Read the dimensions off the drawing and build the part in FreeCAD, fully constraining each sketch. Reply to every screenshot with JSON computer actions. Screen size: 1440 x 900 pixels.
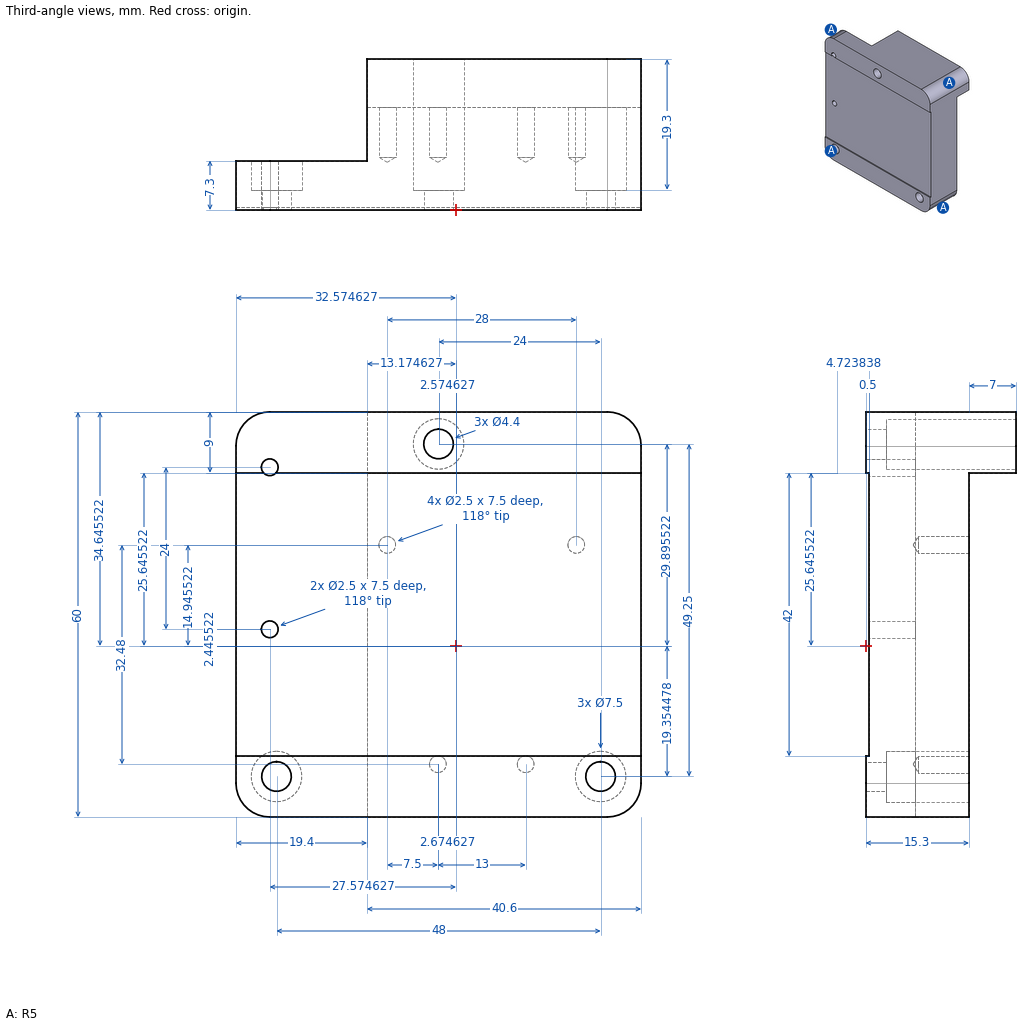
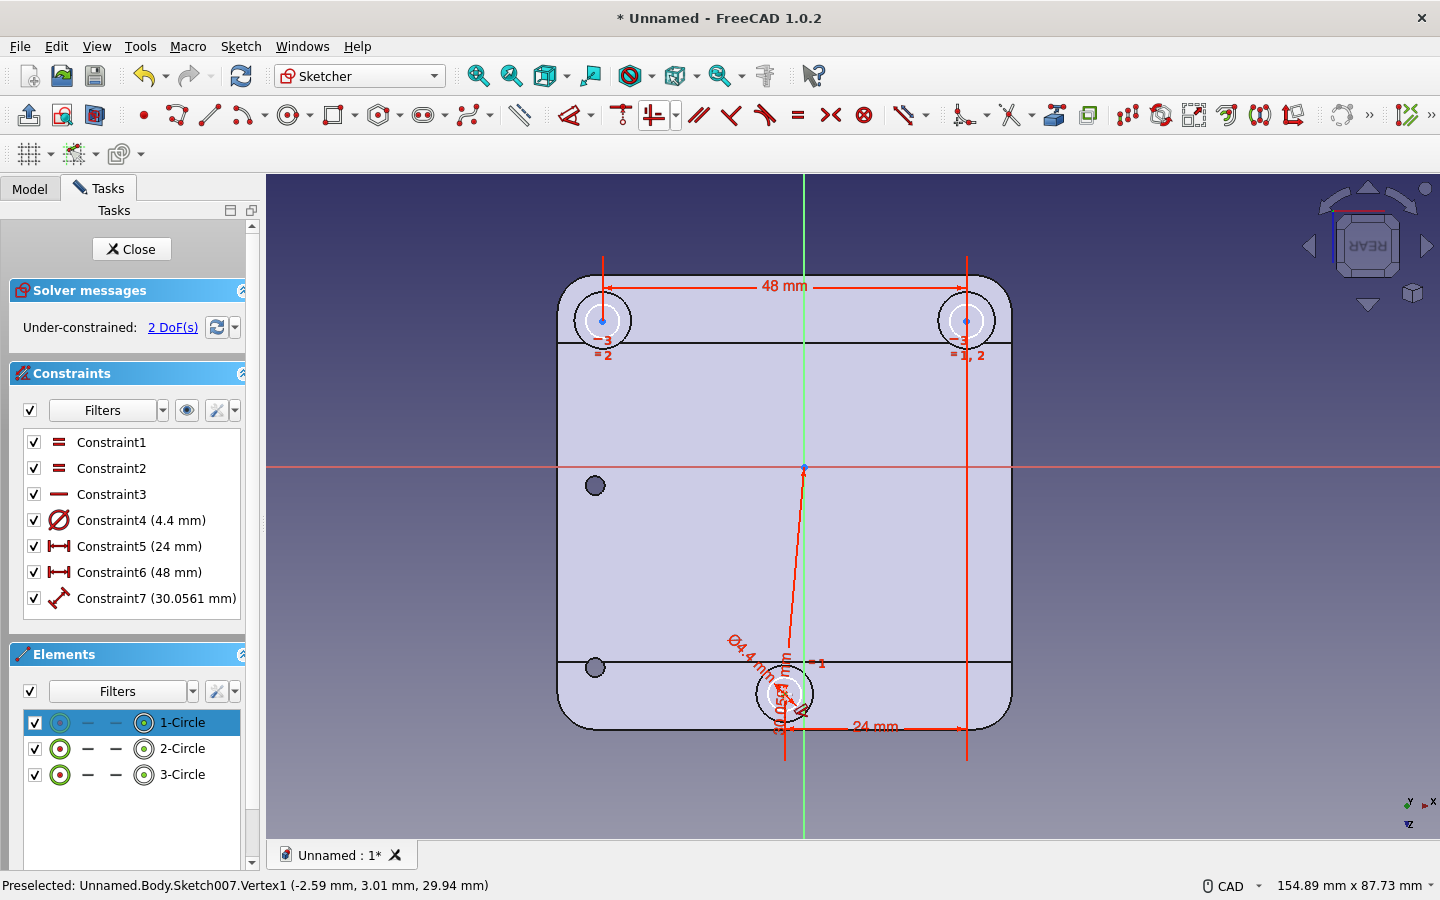
{"action": "left_click", "coordinate": [967, 321]}
{"action": "left_click", "coordinate": [1001, 508]}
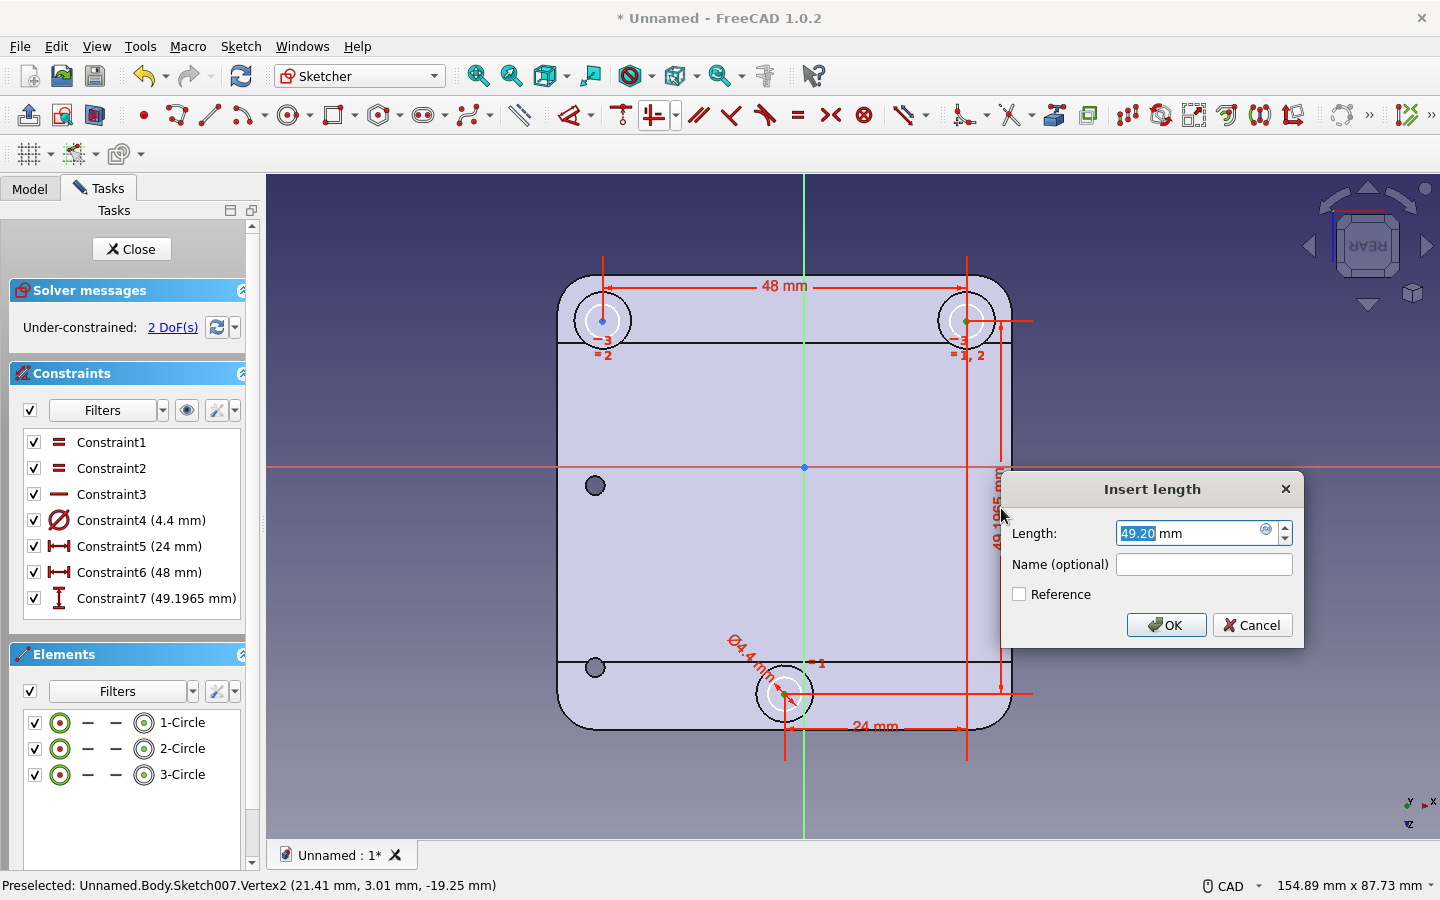
{"action": "type", "text": "49.25"}
{"action": "key", "text": "Return"}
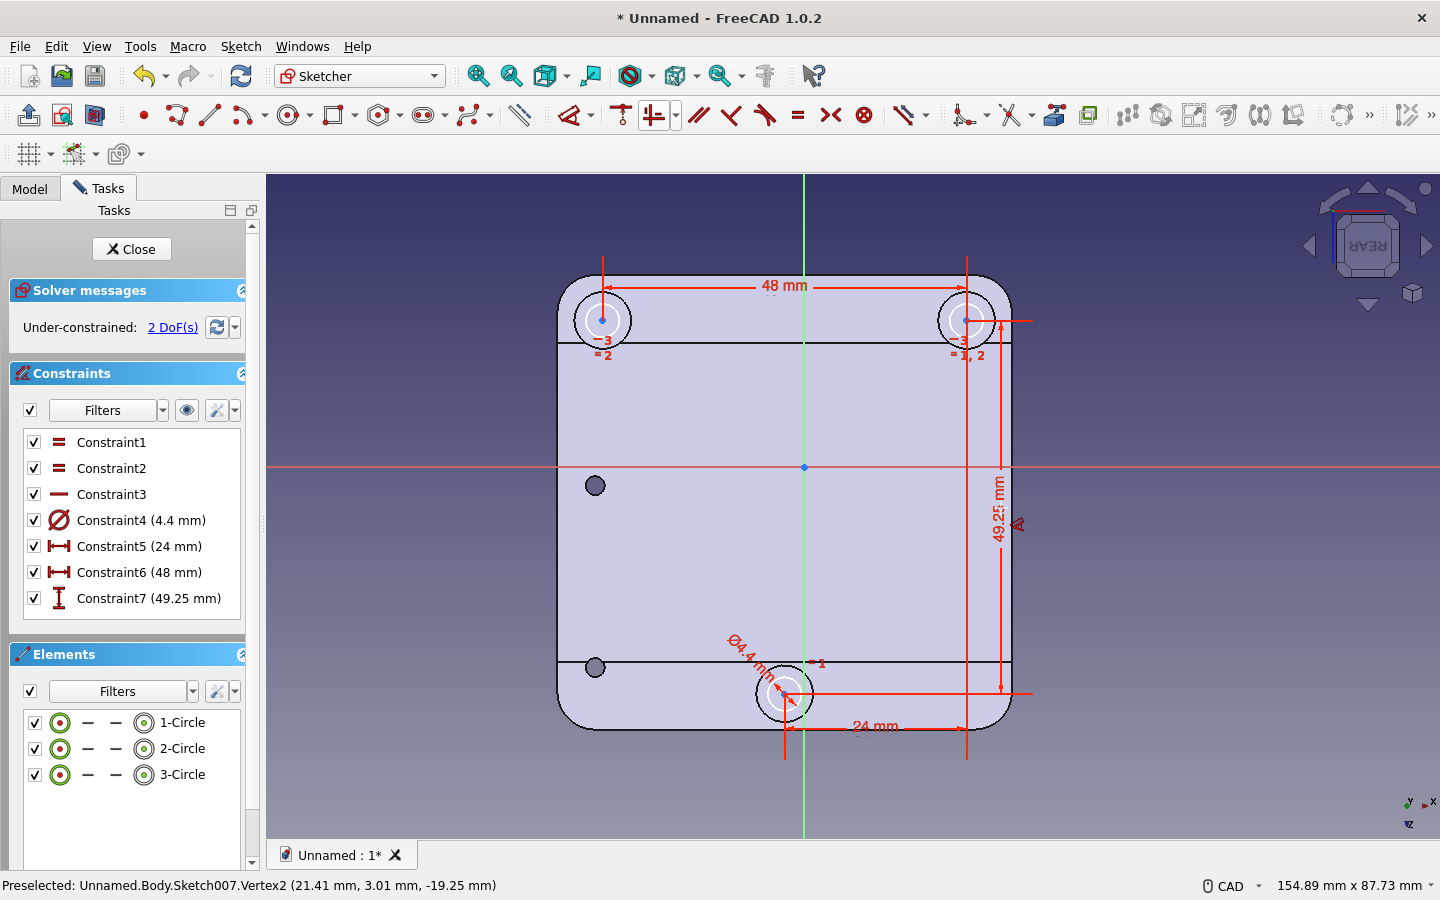
{"action": "scroll", "coordinate": [785, 694], "scroll_direction": "up", "scroll_amount": 4}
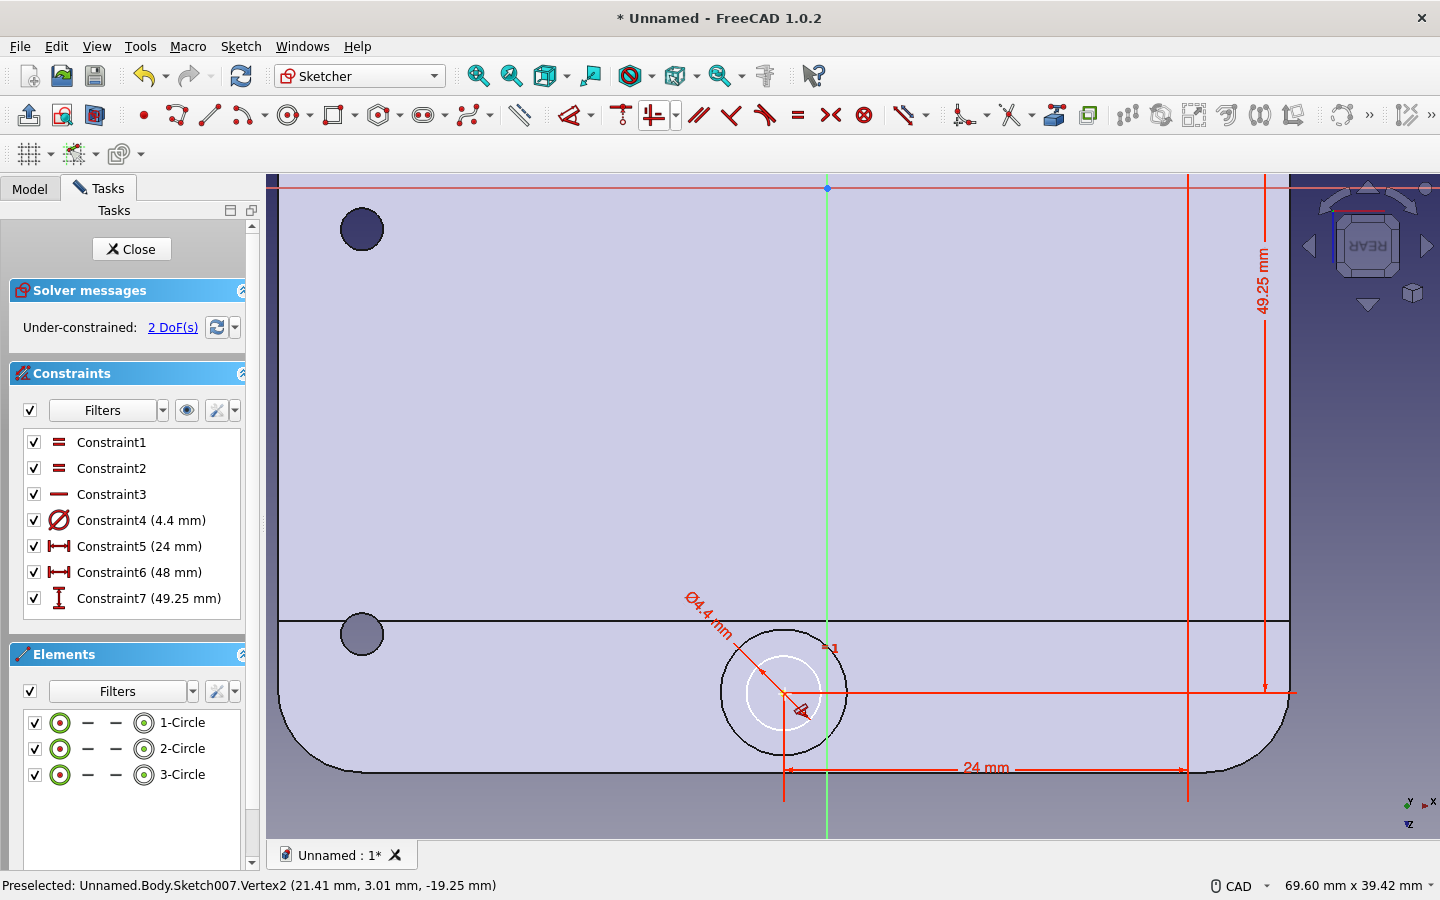
{"action": "left_click", "coordinate": [784, 693]}
{"action": "left_click", "coordinate": [805, 751]}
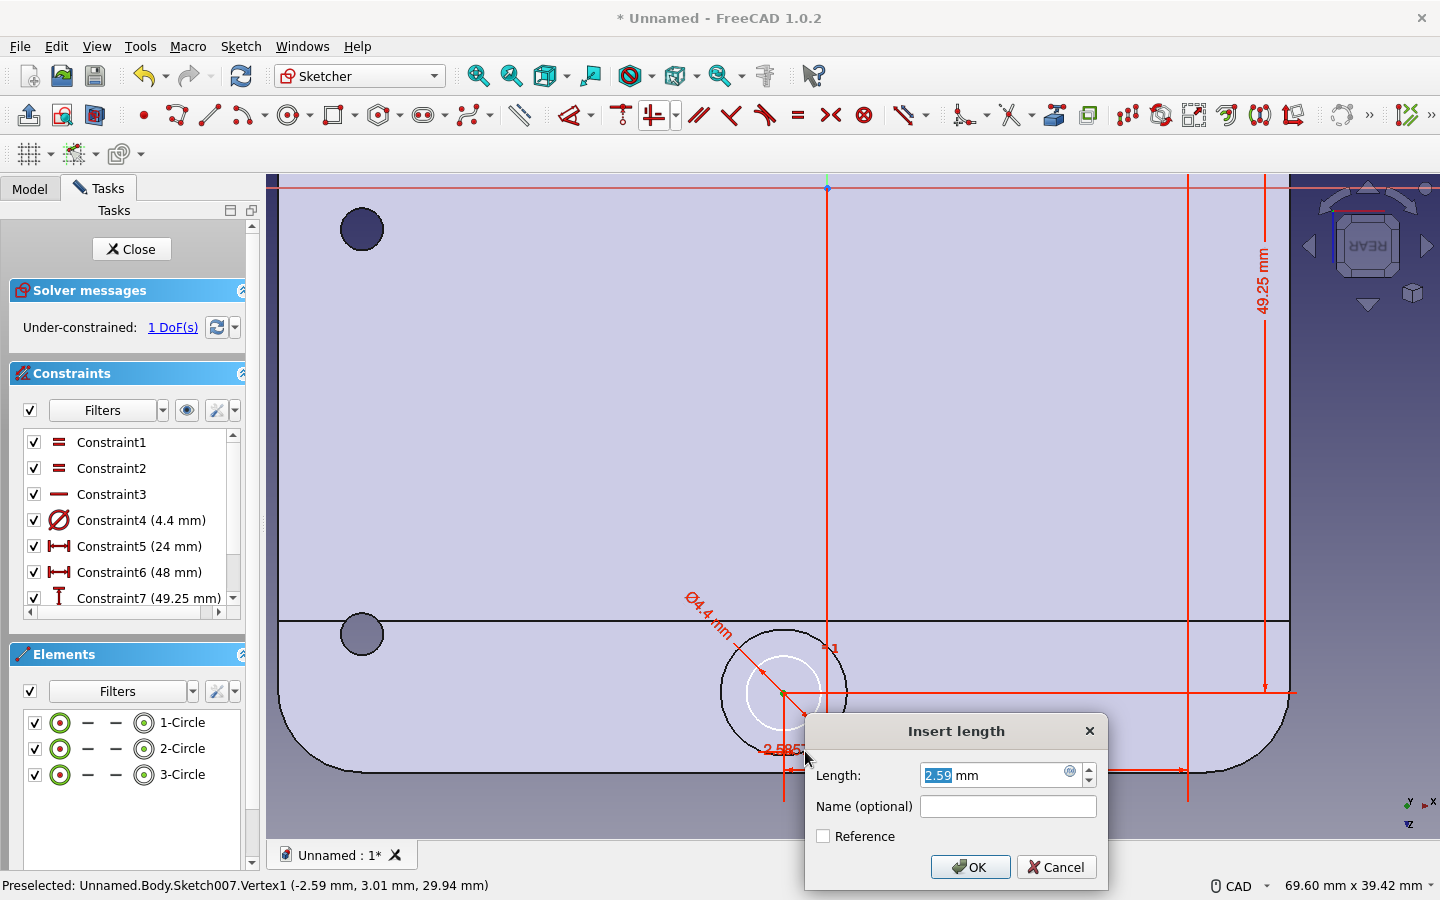
{"action": "type", "text": "2.574627"}
{"action": "key", "text": "Return"}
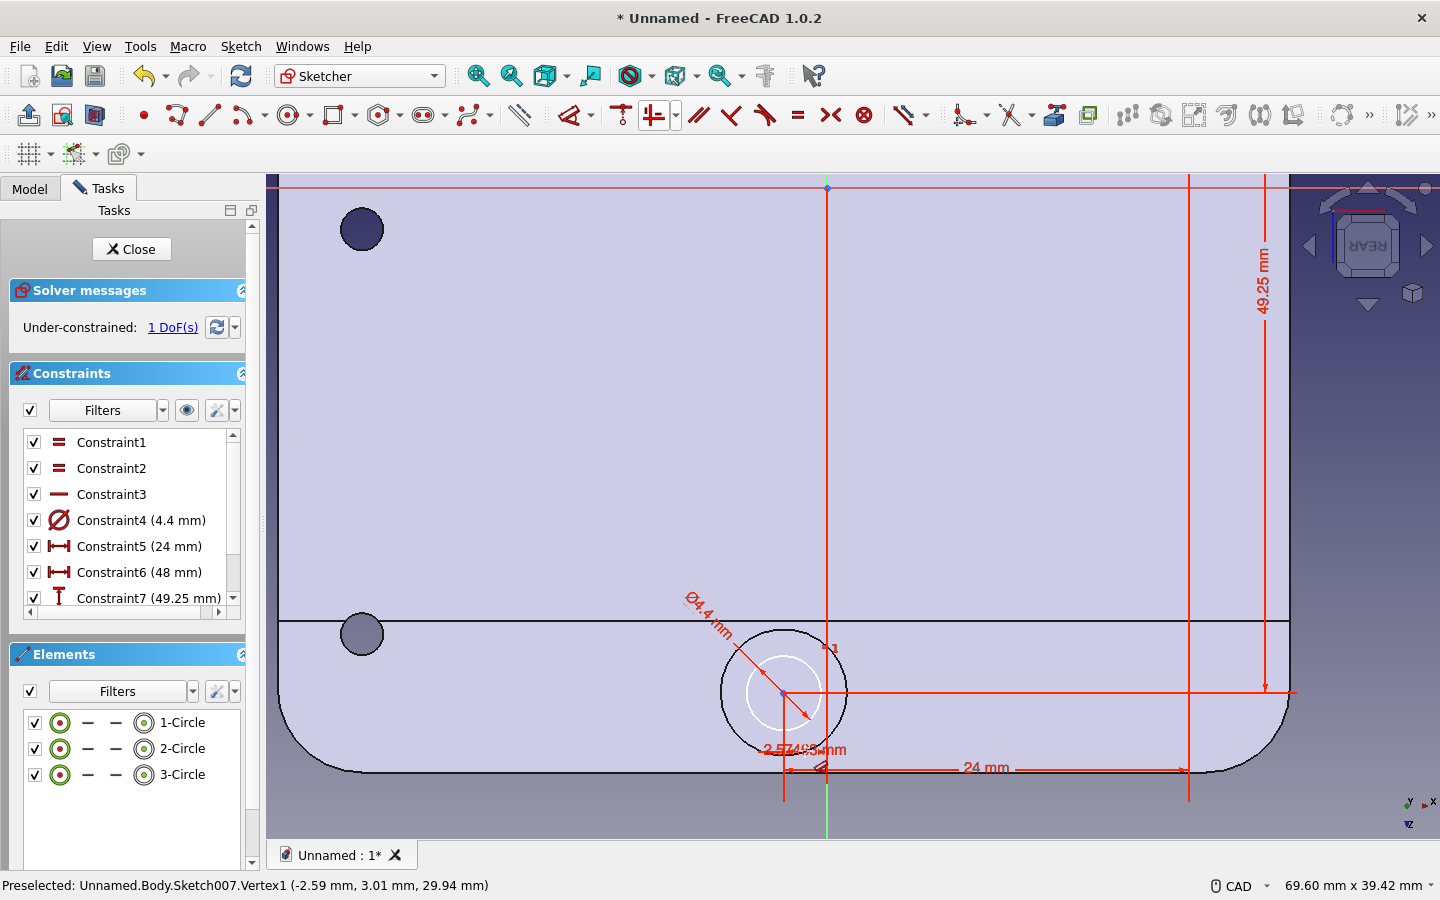
{"action": "left_click", "coordinate": [784, 693]}
{"action": "left_click", "coordinate": [861, 448]}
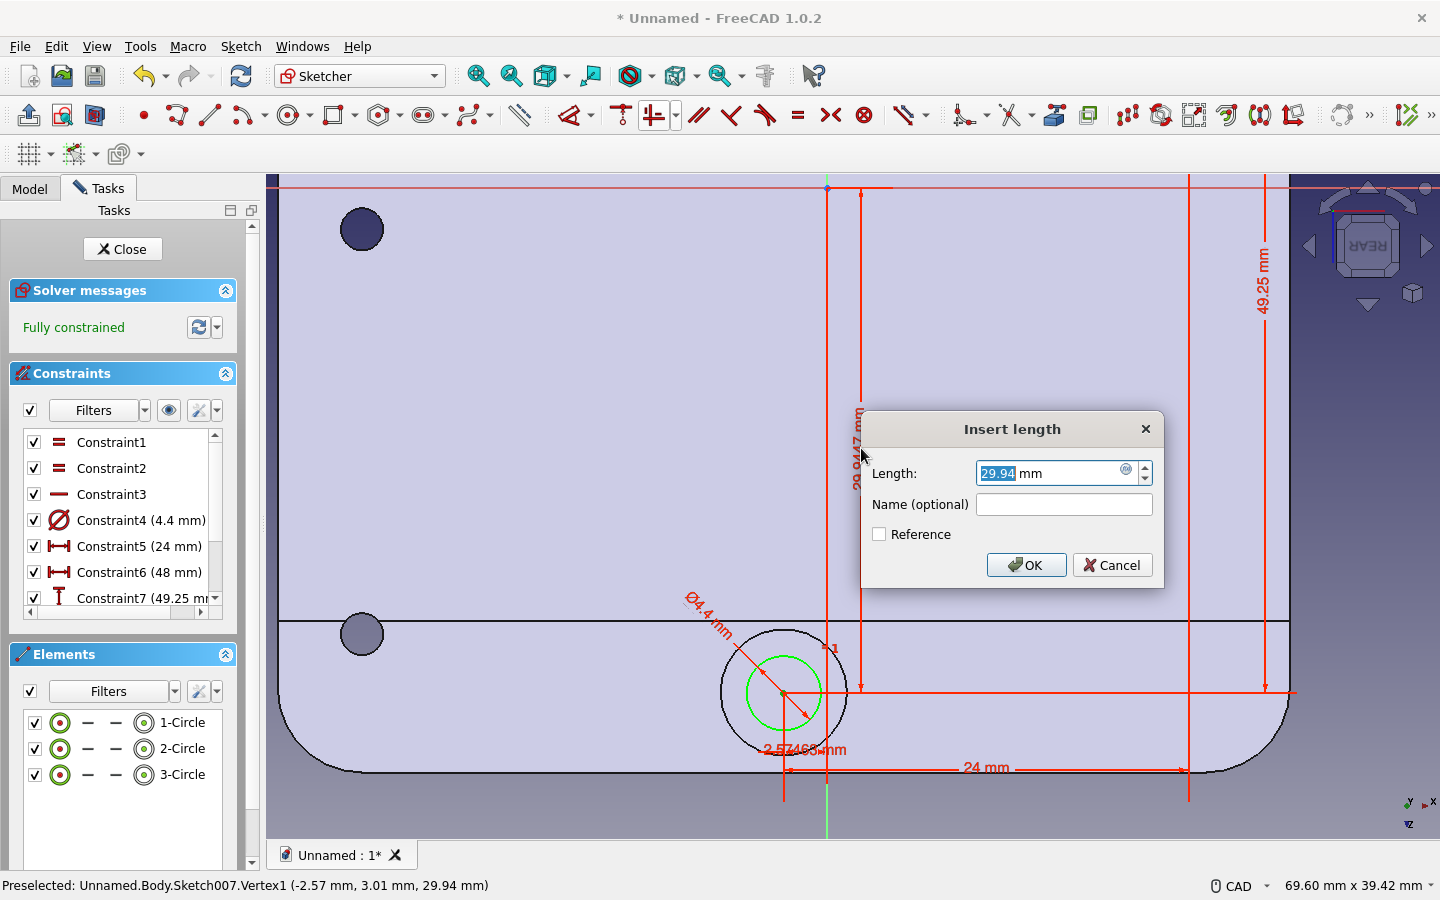
{"action": "type", "text": "29.895522"}
{"action": "key", "text": "Return"}
{"action": "key", "text": "Escape"}